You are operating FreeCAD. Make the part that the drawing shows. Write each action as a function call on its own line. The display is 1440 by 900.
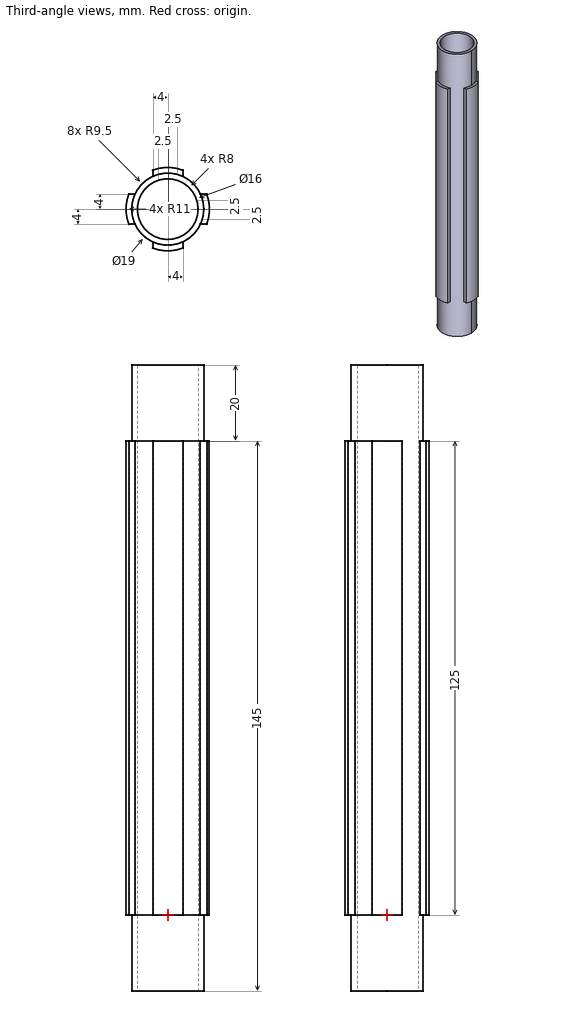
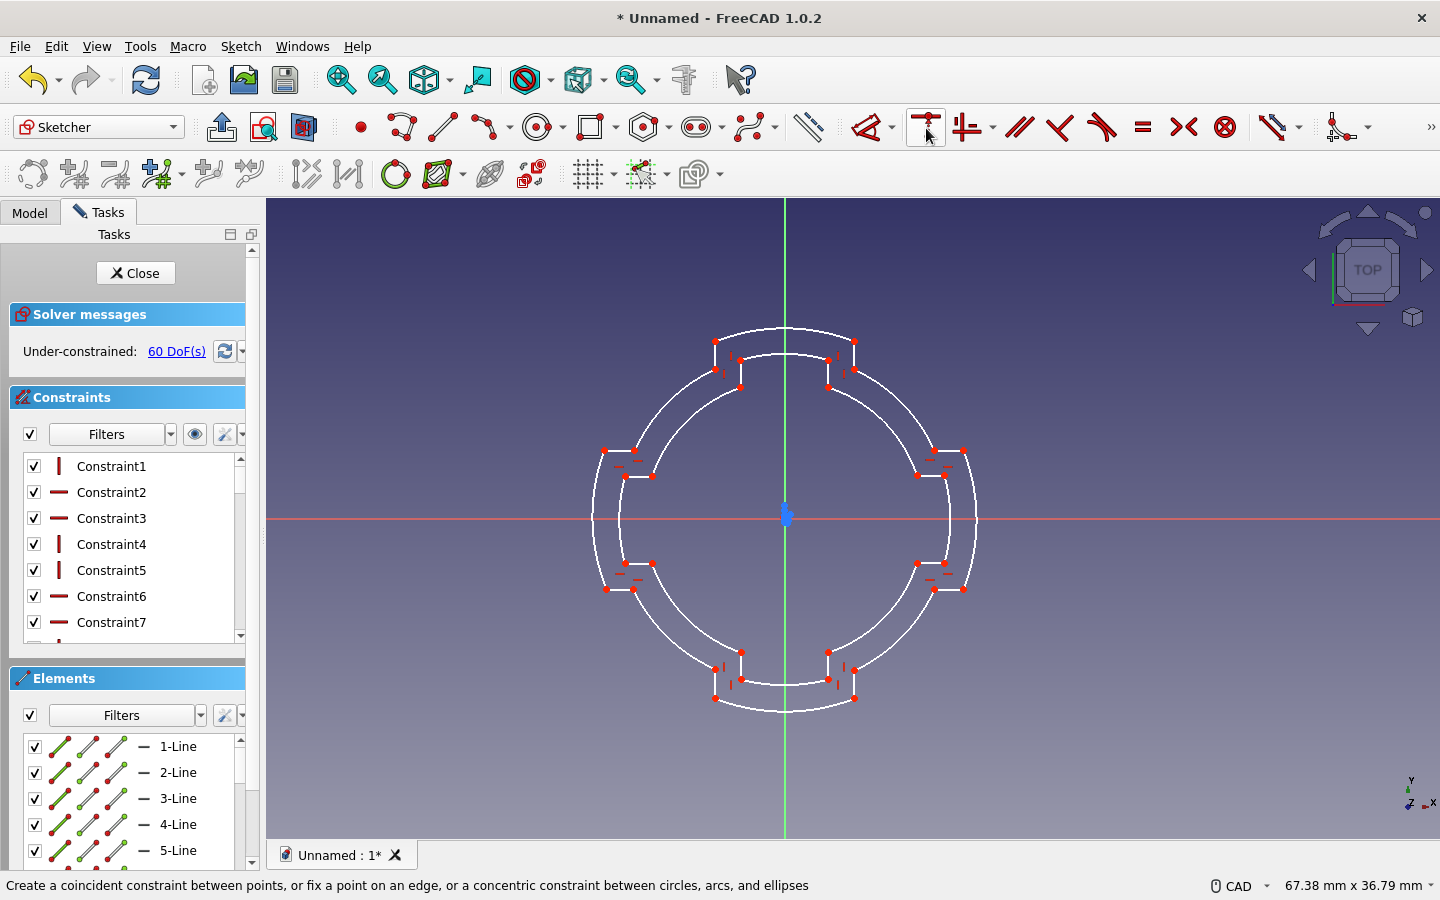
click(685, 387)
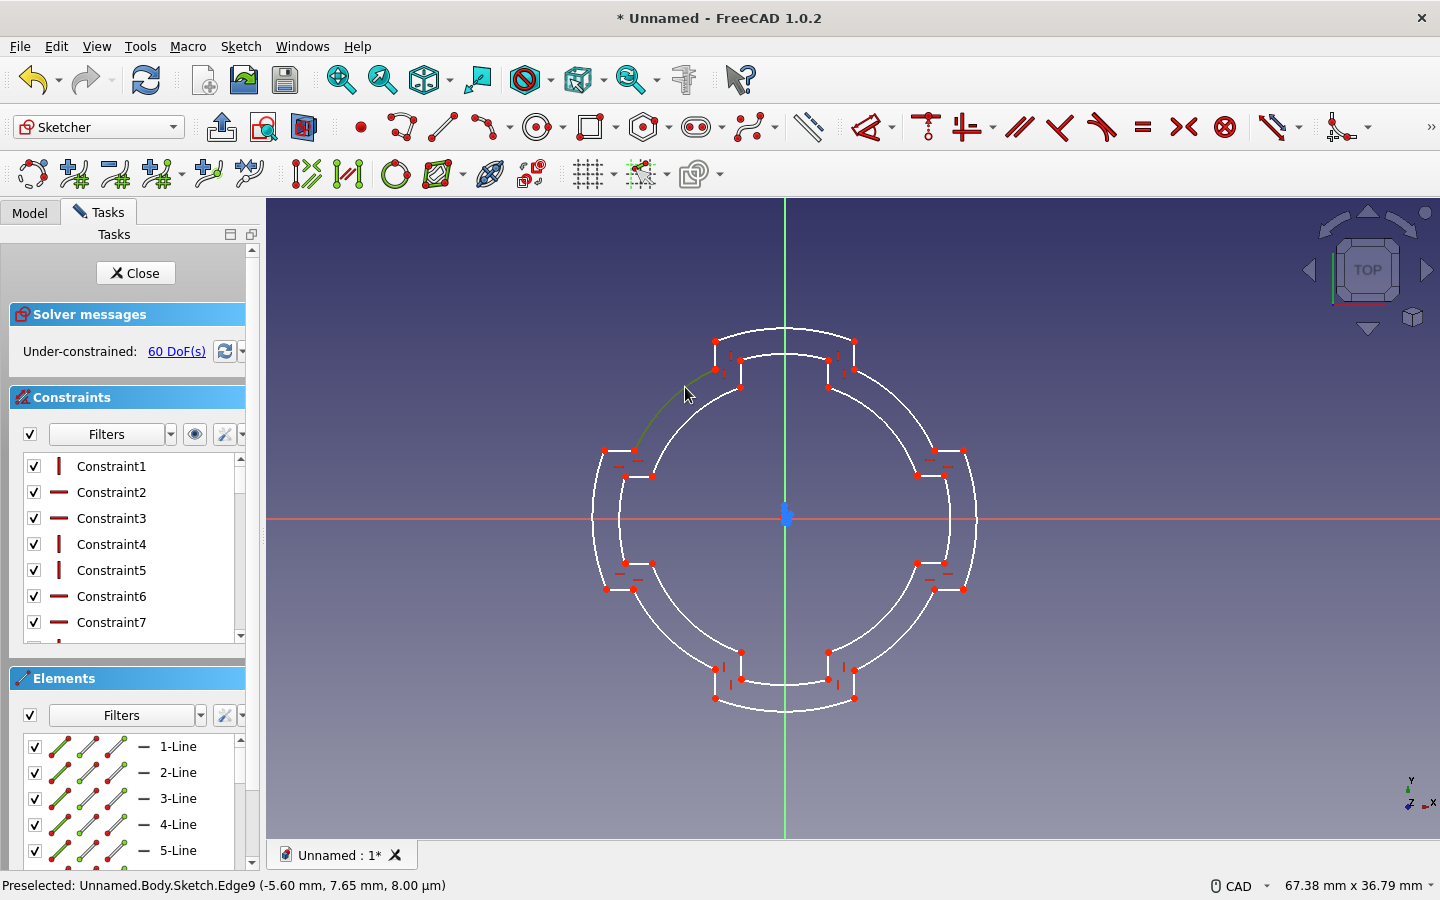
click(756, 710)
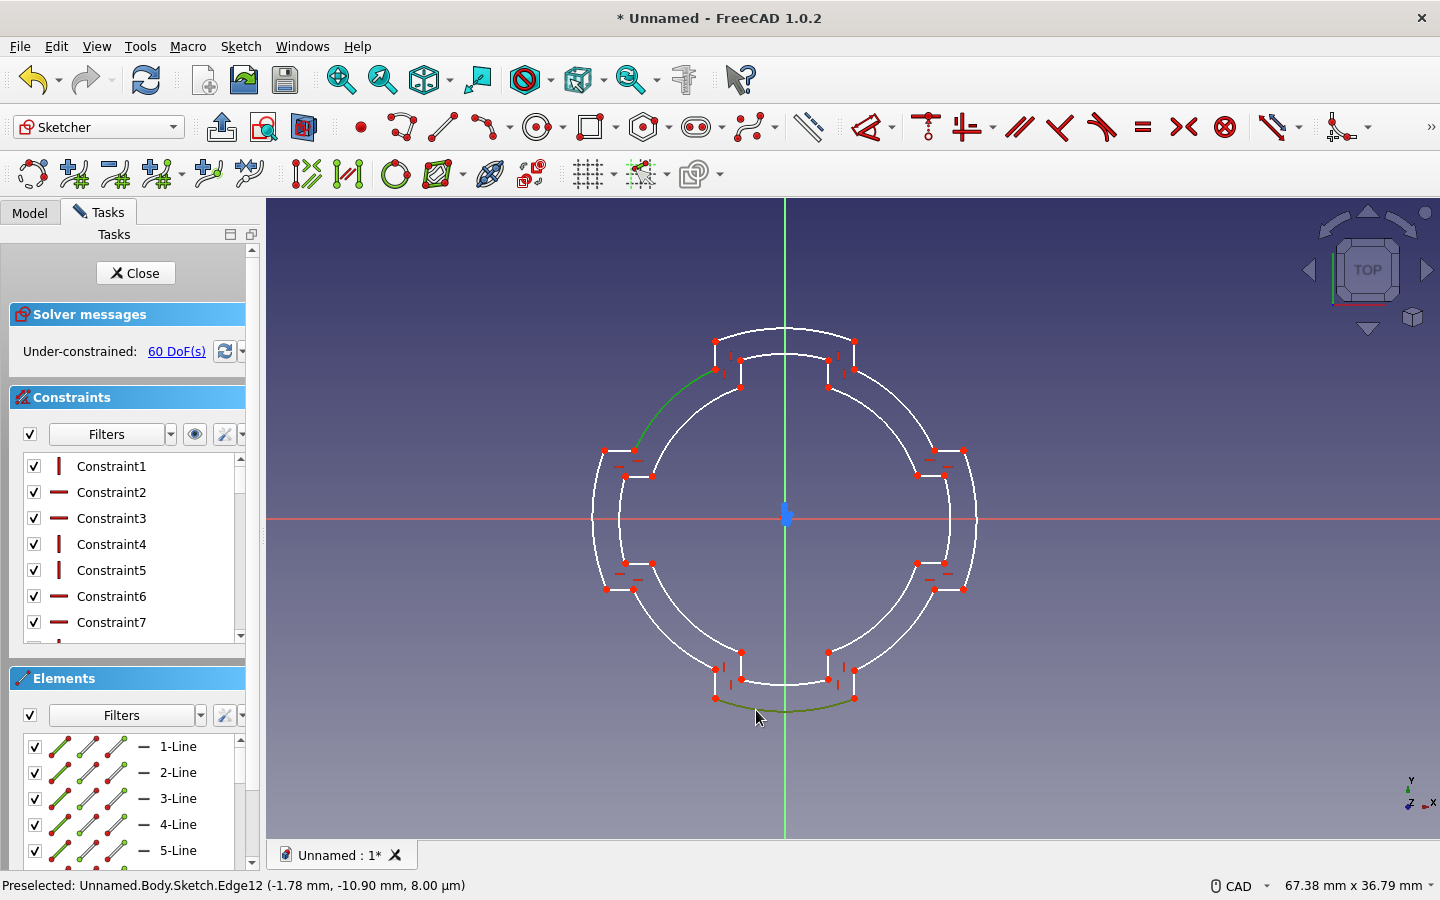
click(926, 128)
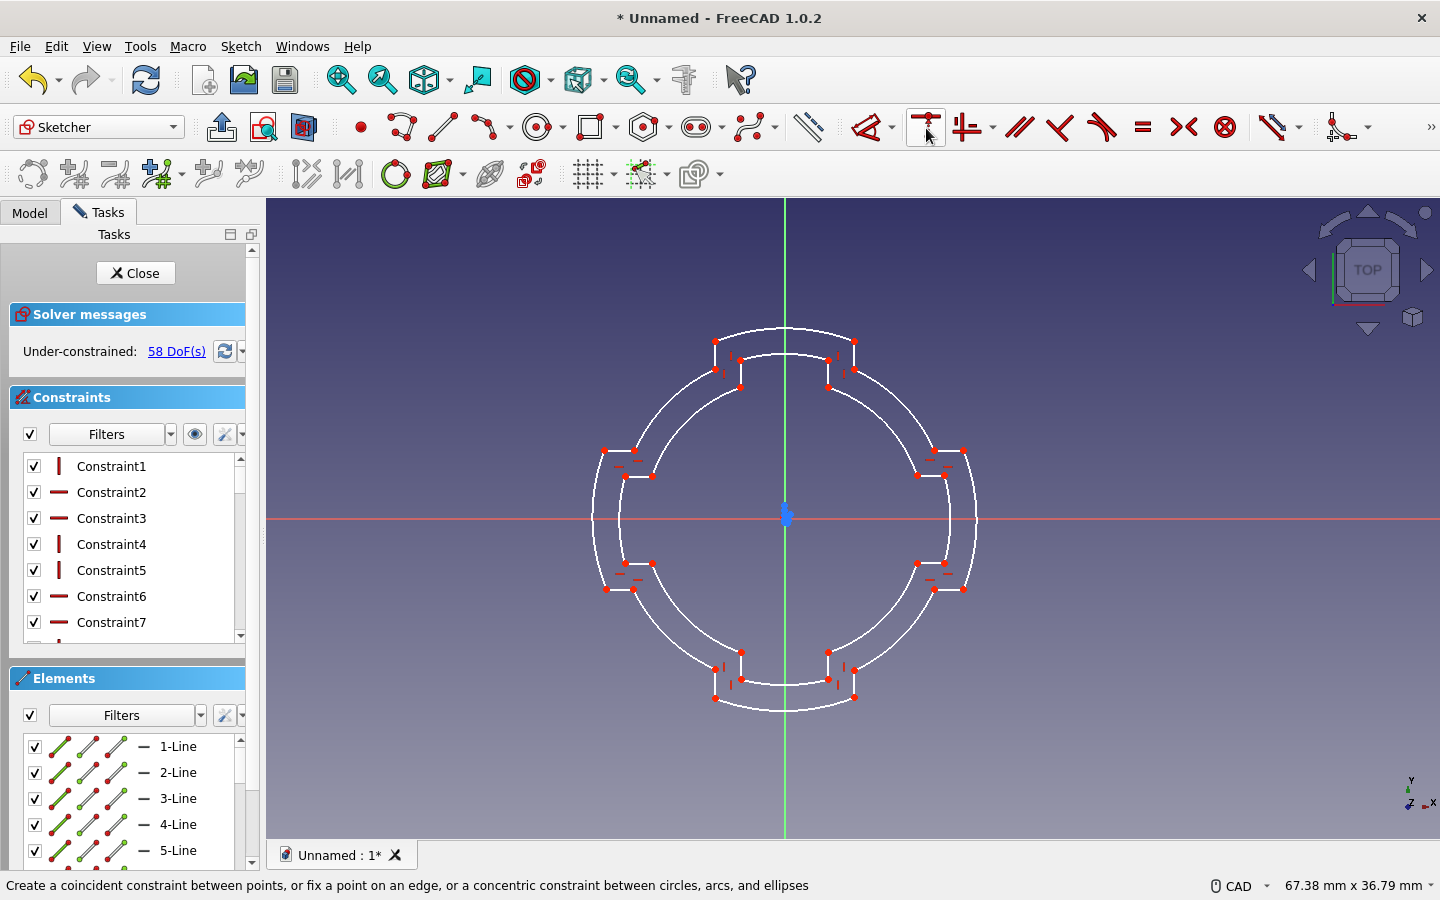
click(685, 387)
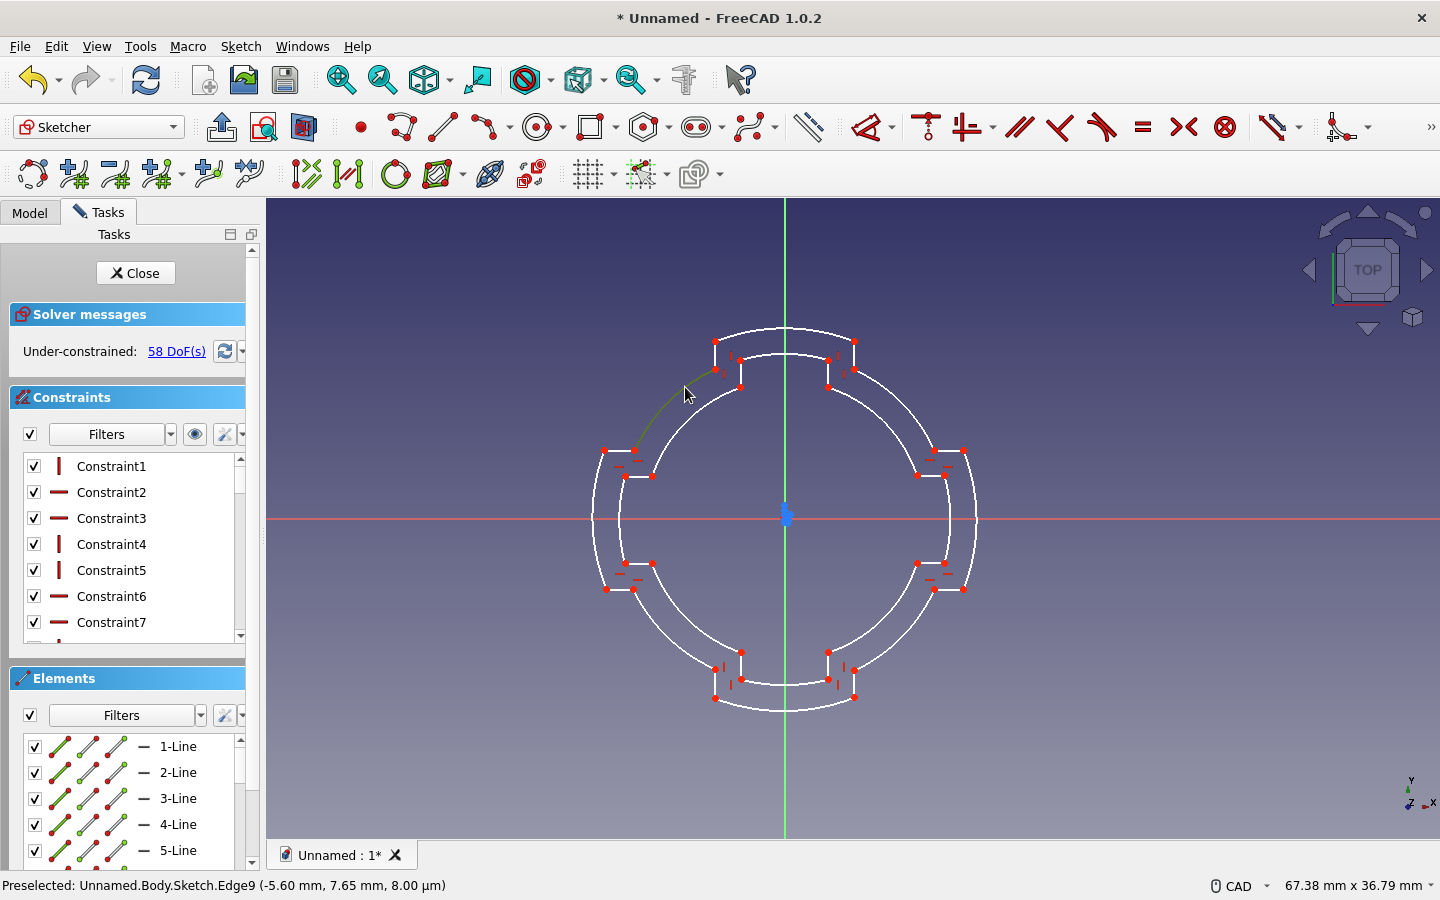
click(884, 653)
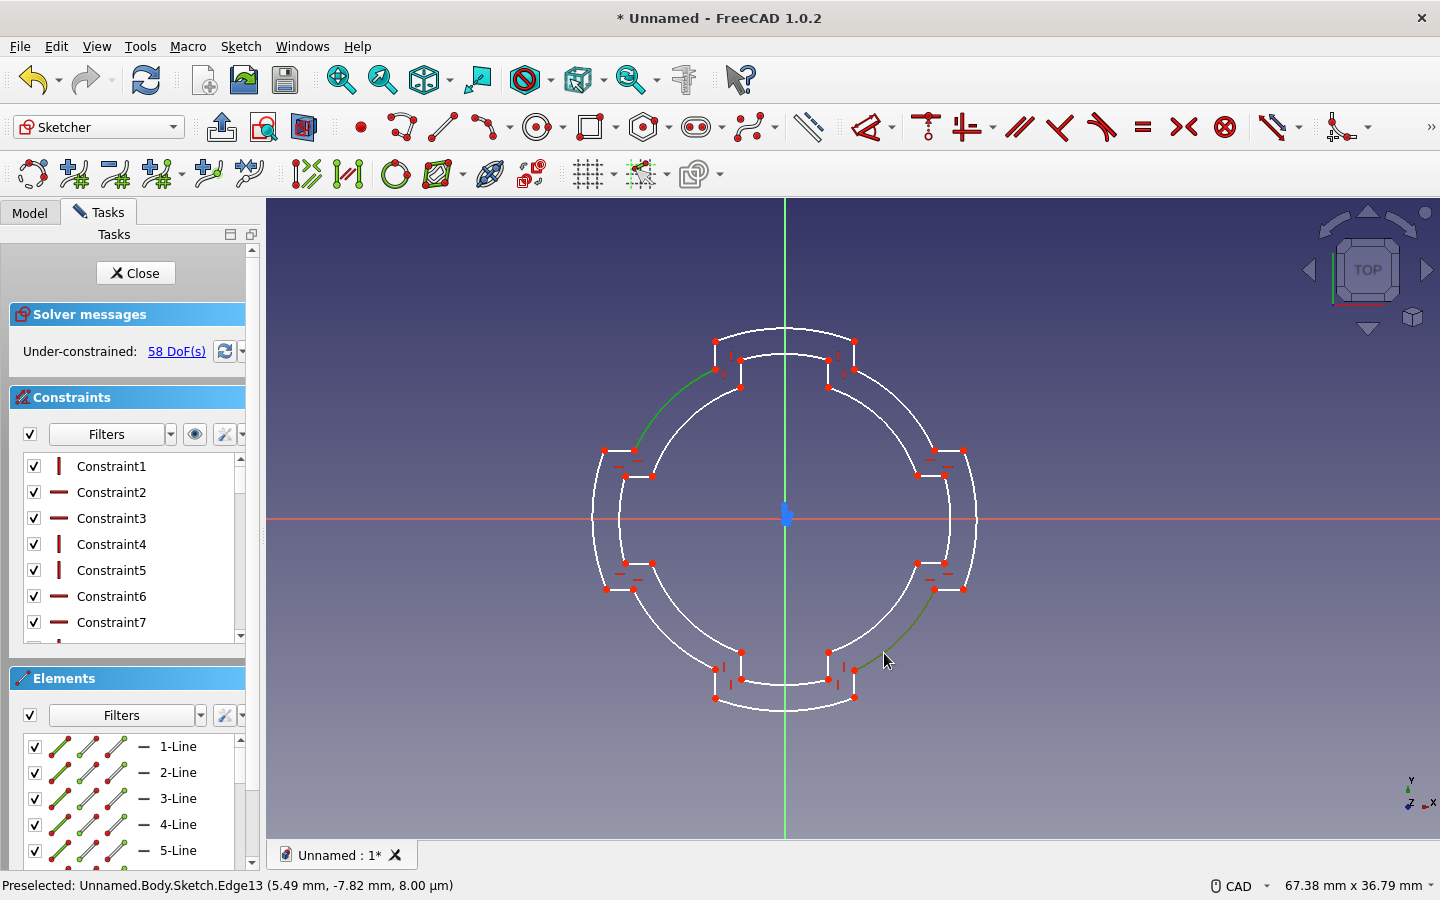
click(926, 128)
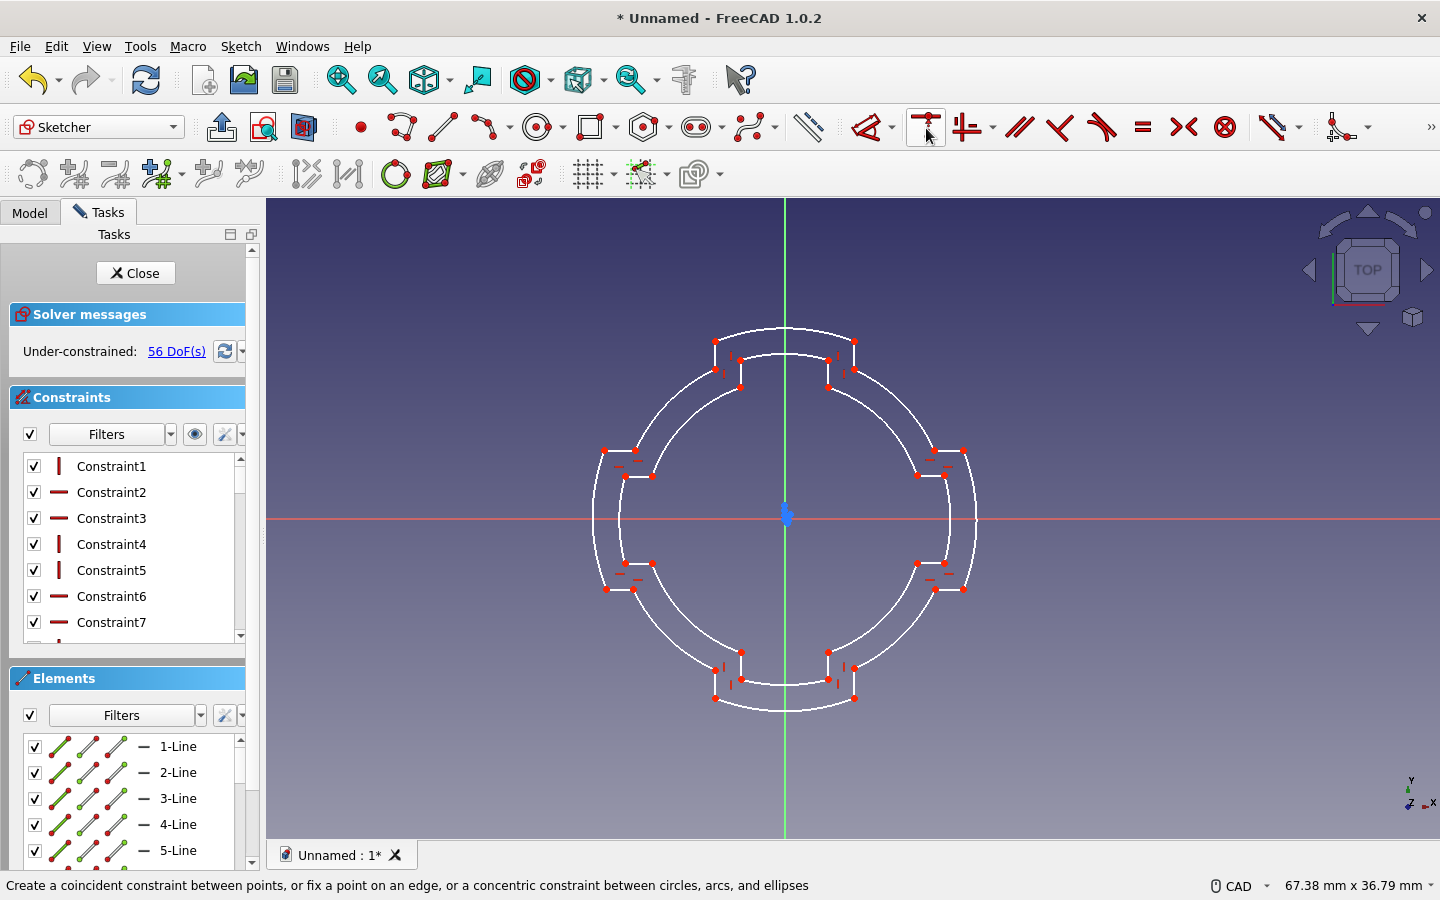
click(686, 387)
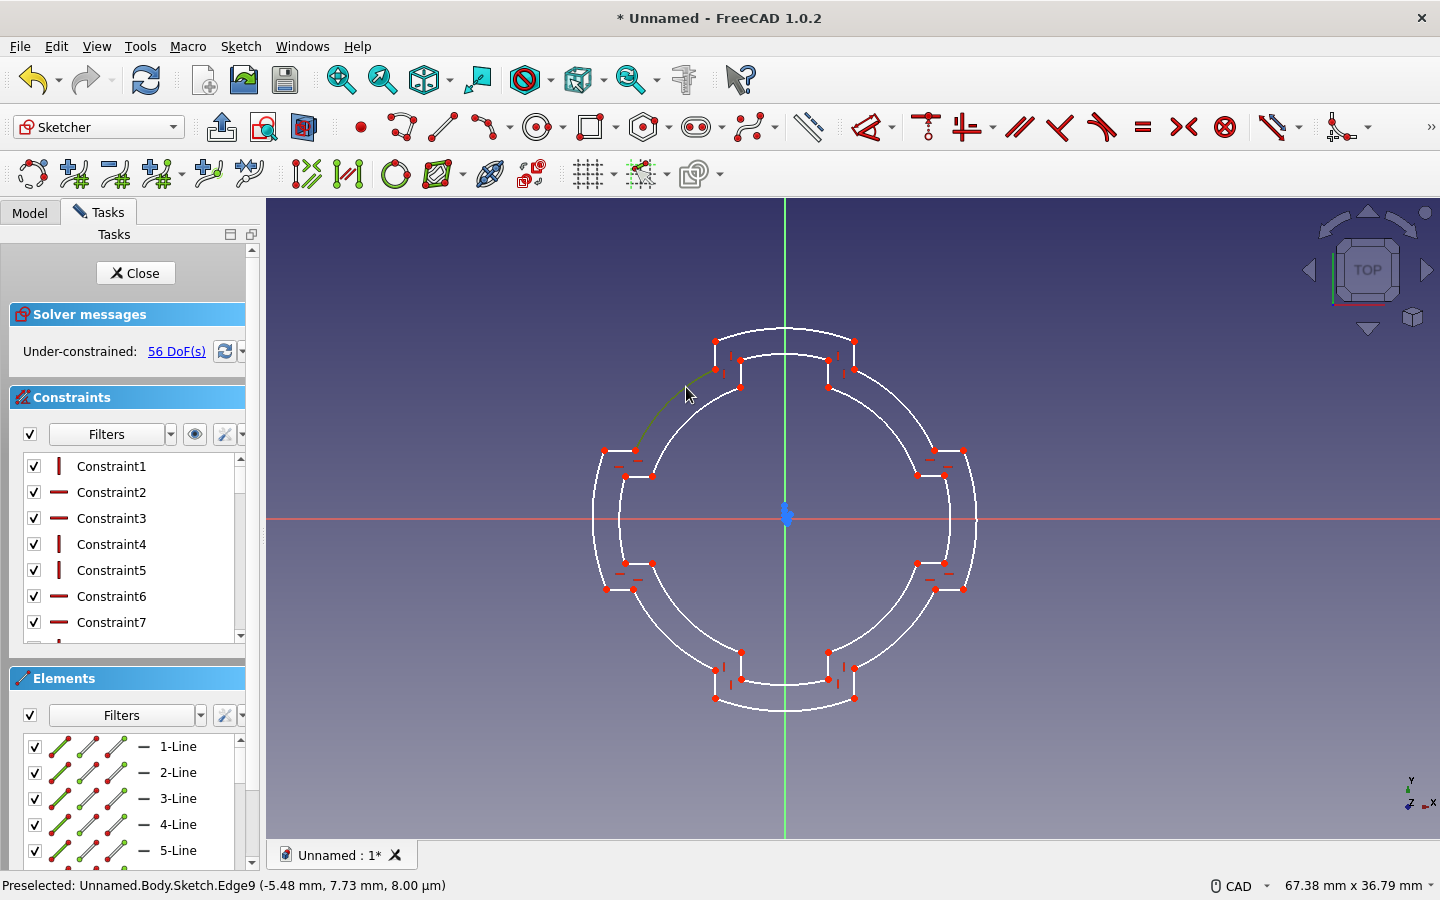
click(974, 549)